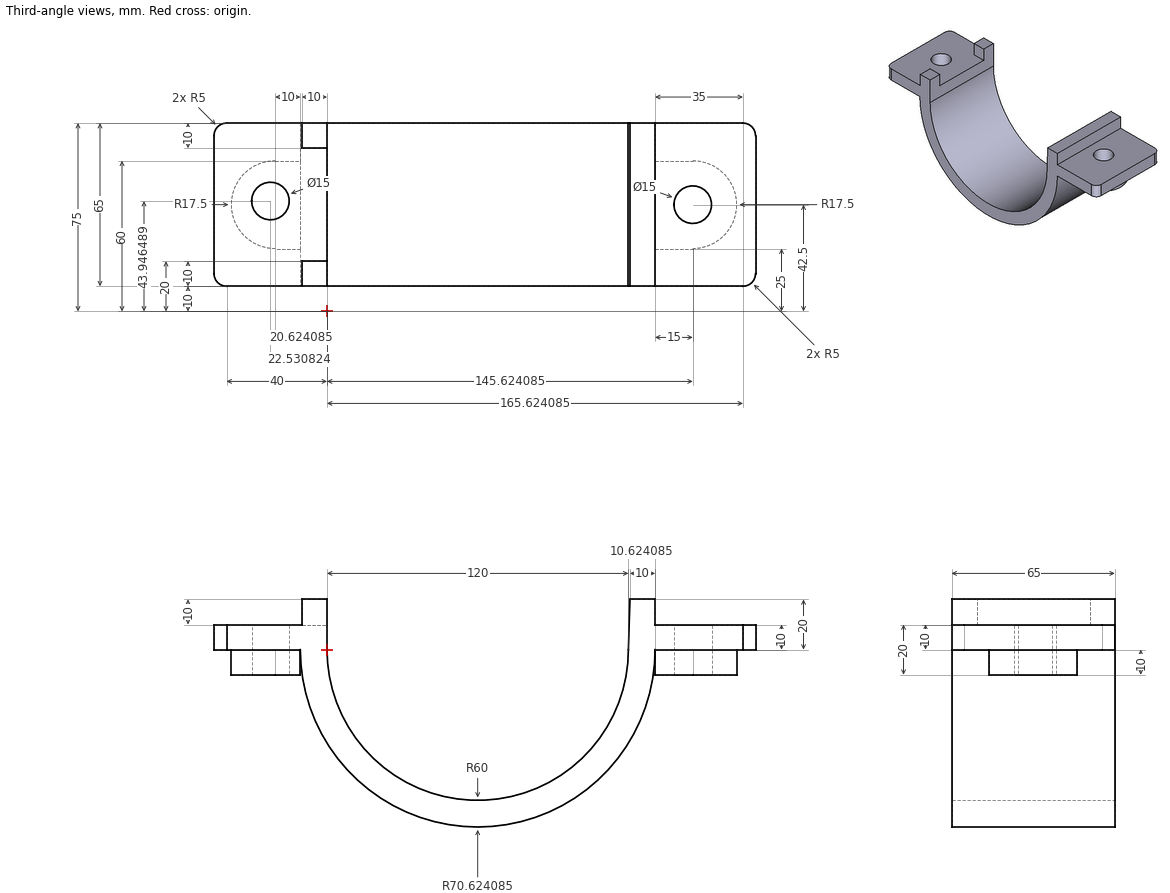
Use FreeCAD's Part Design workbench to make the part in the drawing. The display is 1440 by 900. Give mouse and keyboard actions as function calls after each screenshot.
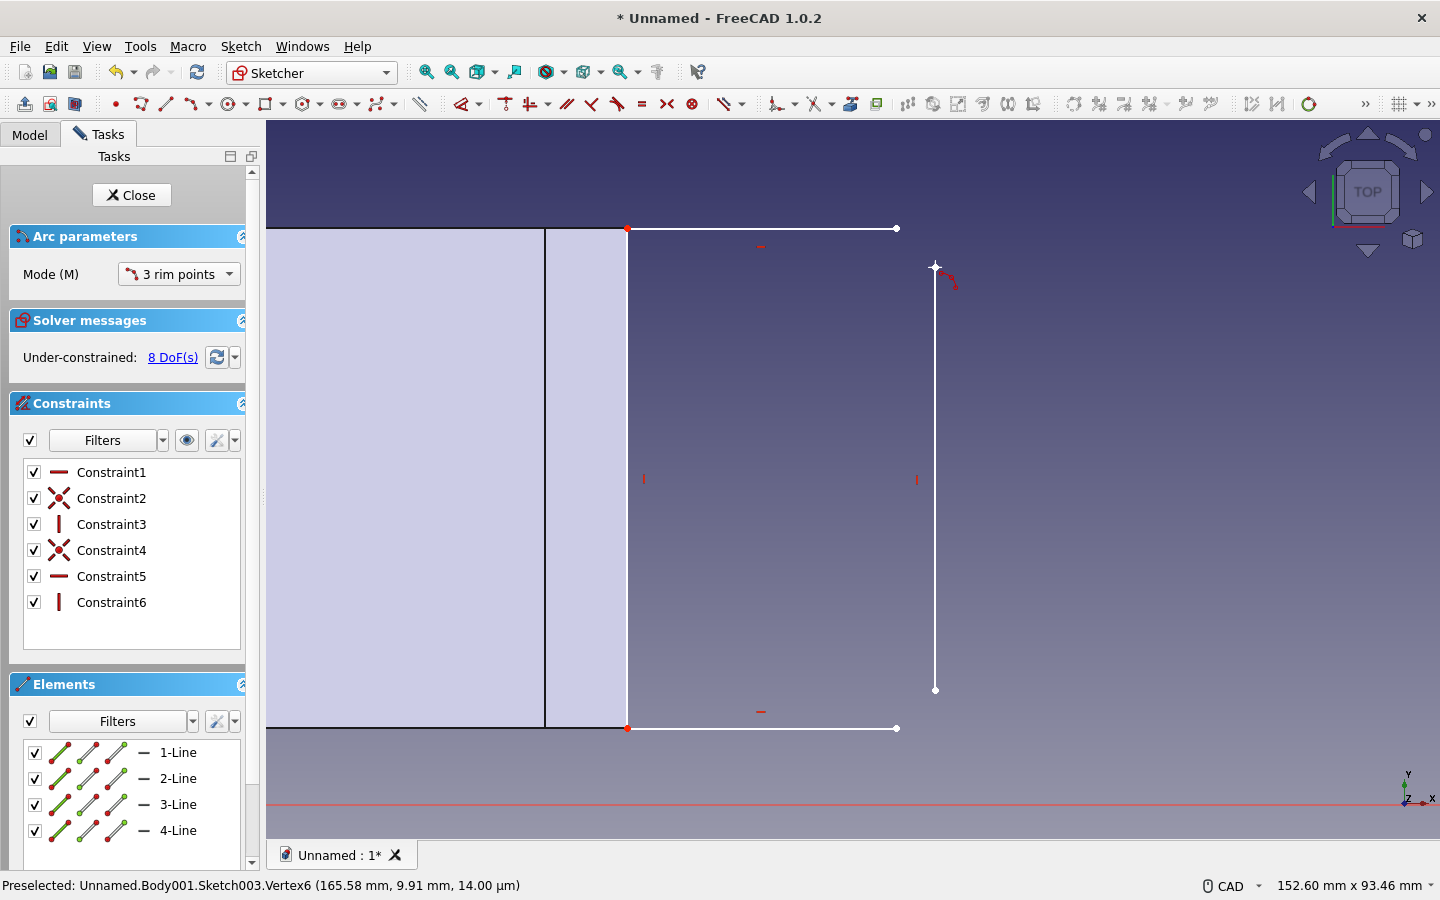
click(896, 729)
click(935, 691)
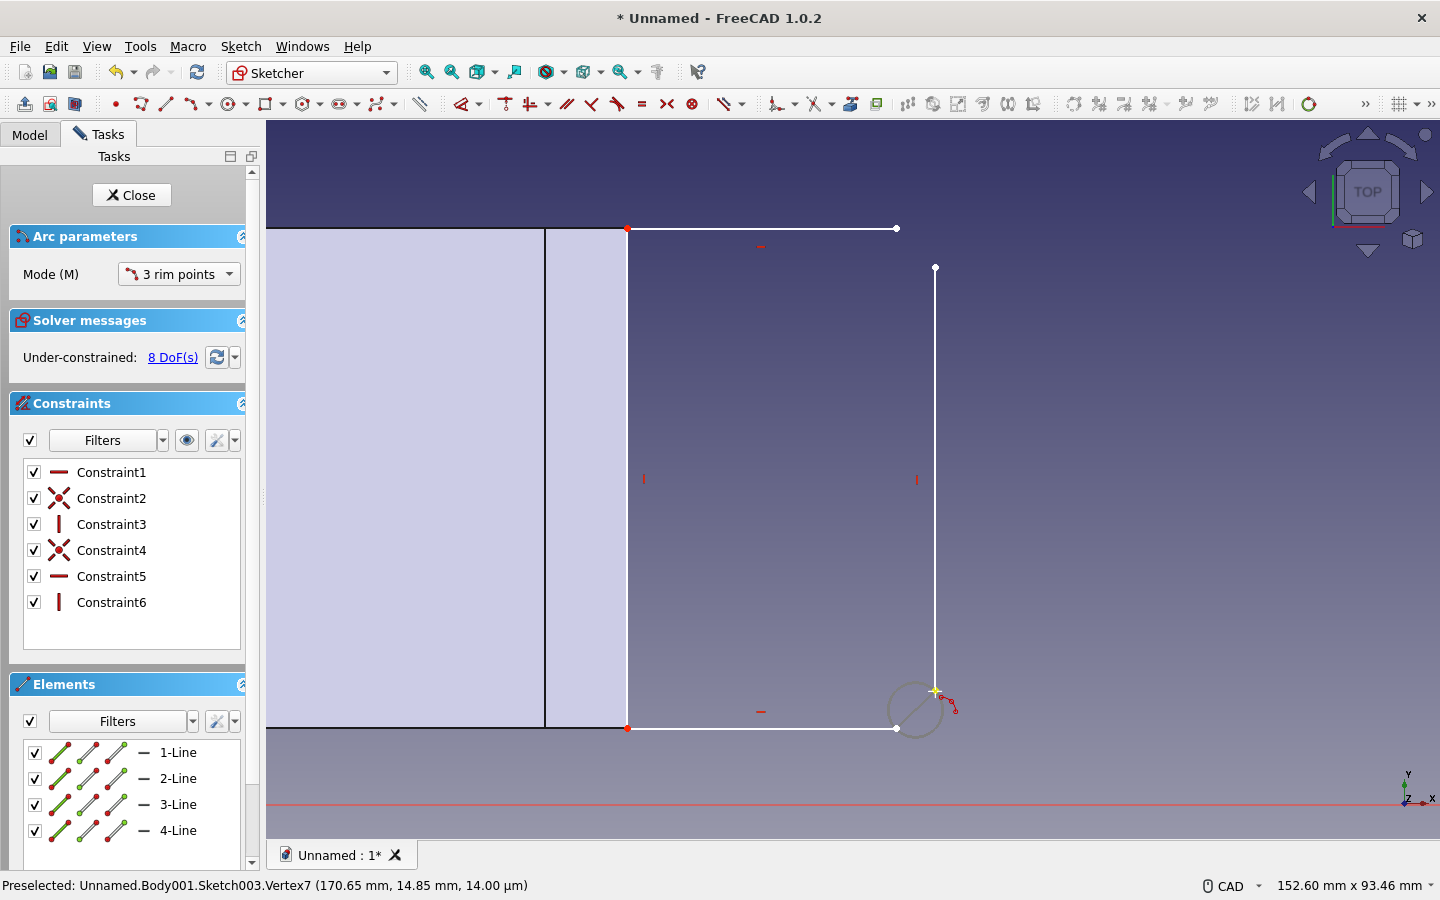
scroll(924, 717, up, 2)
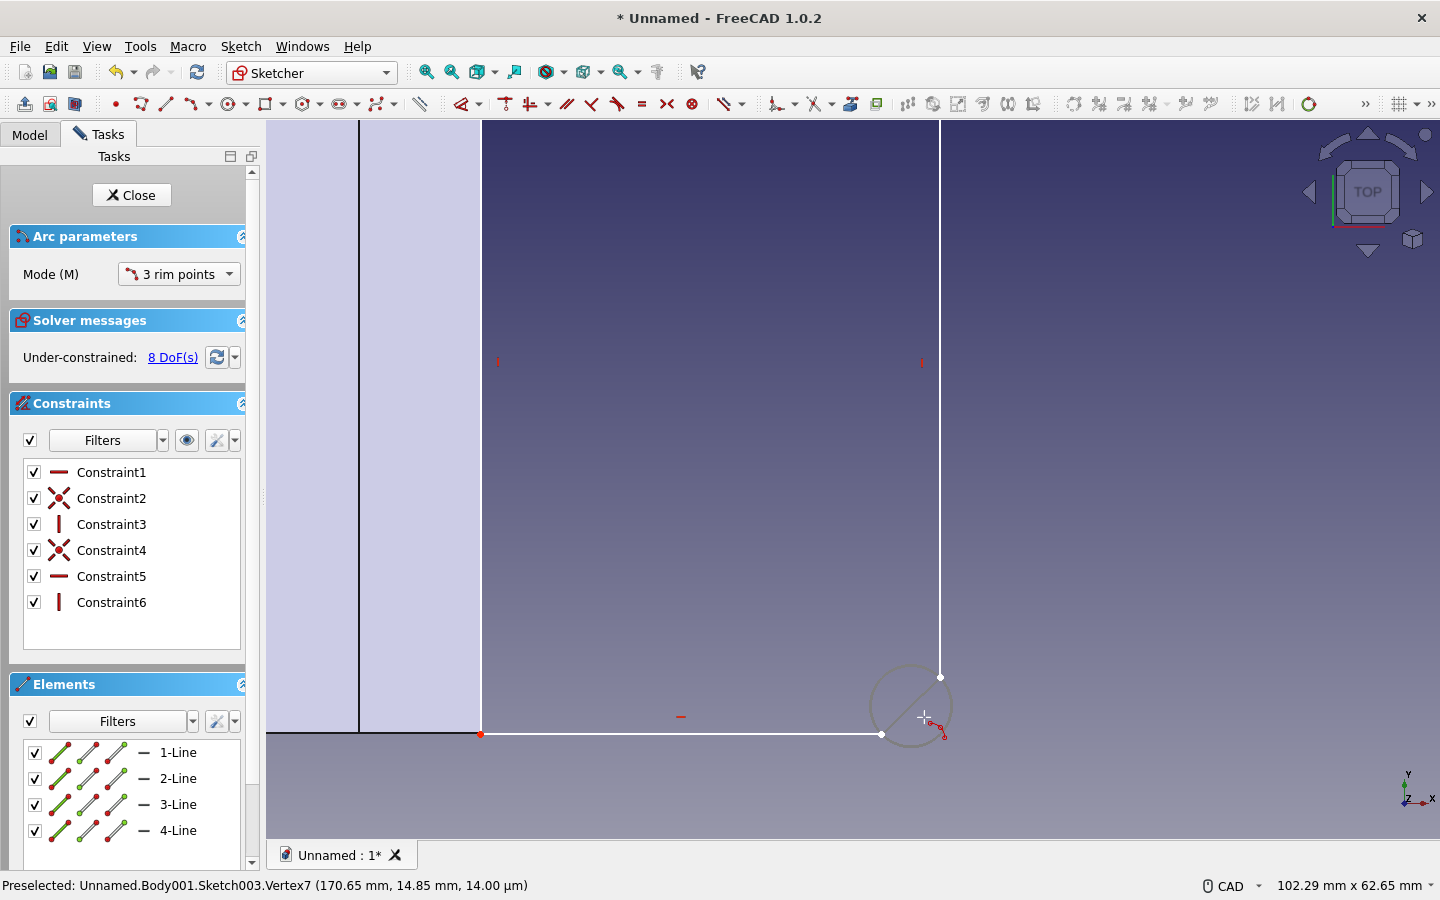
click(923, 717)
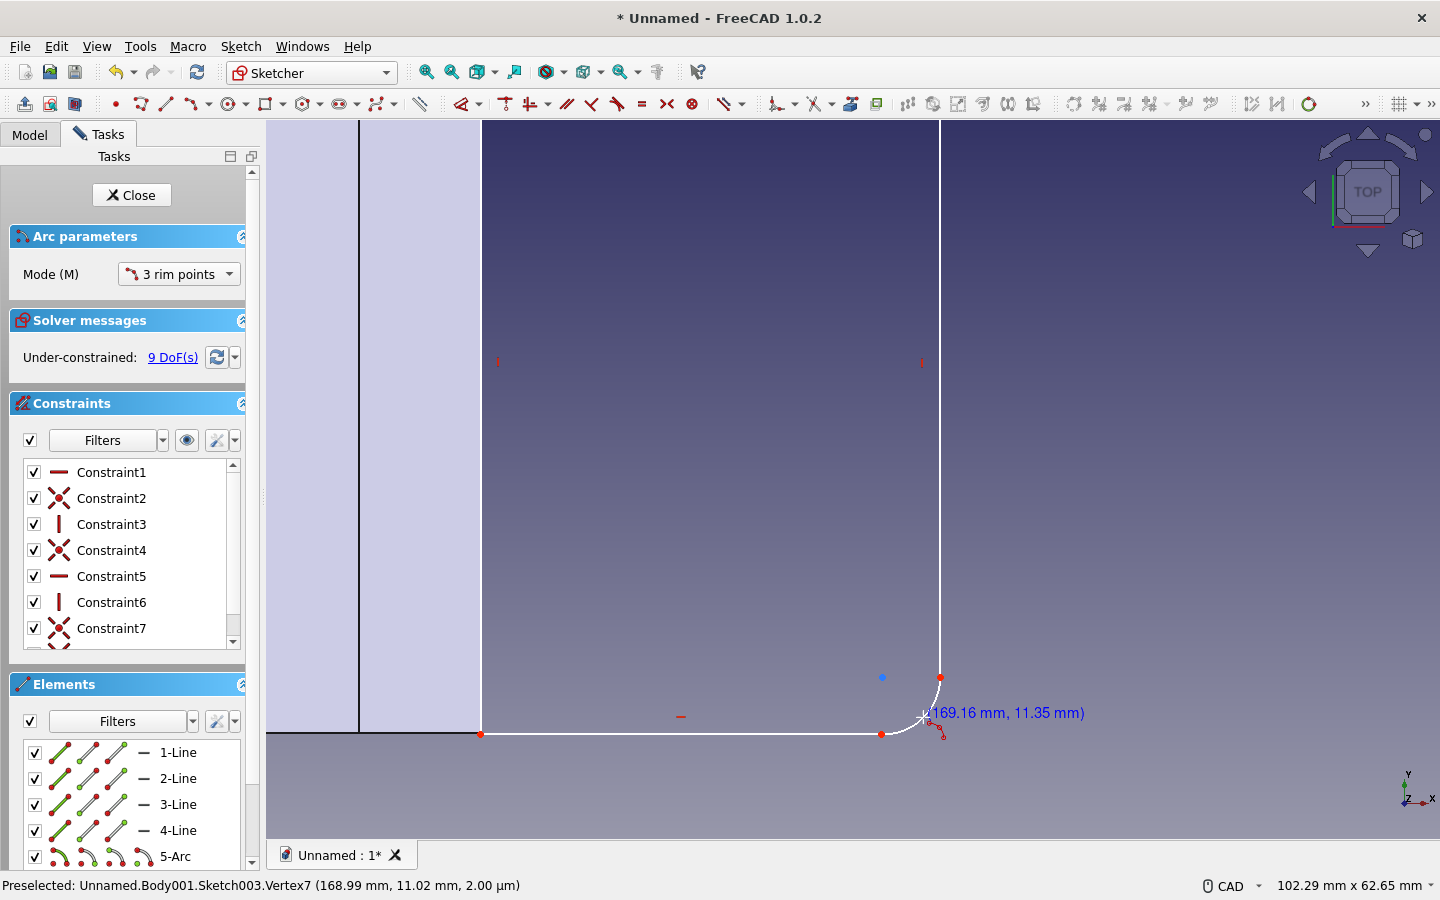
scroll(935, 722, down, 2)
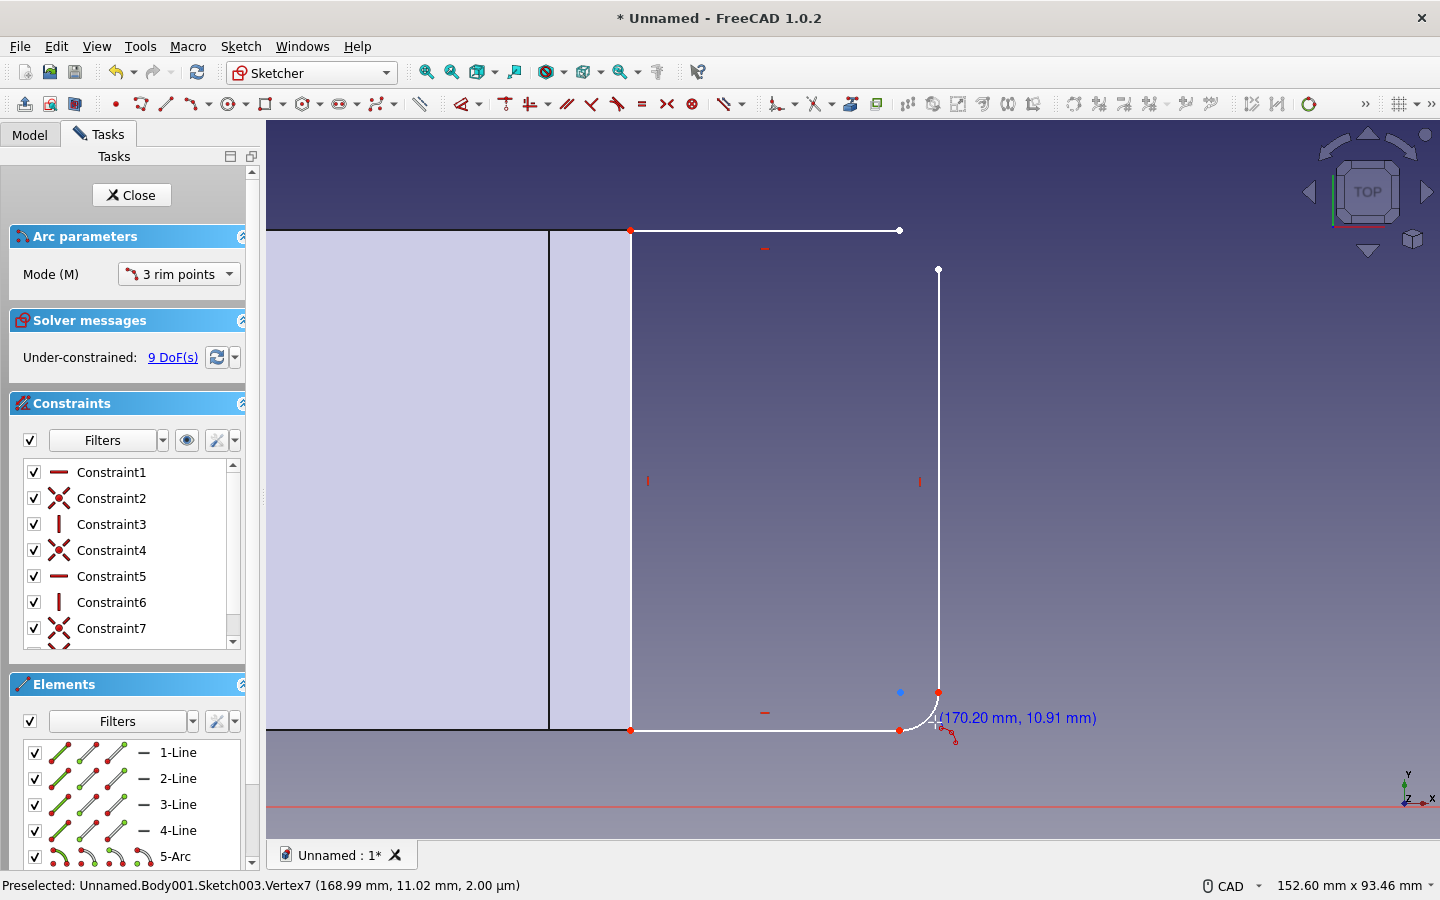
click(939, 270)
click(900, 231)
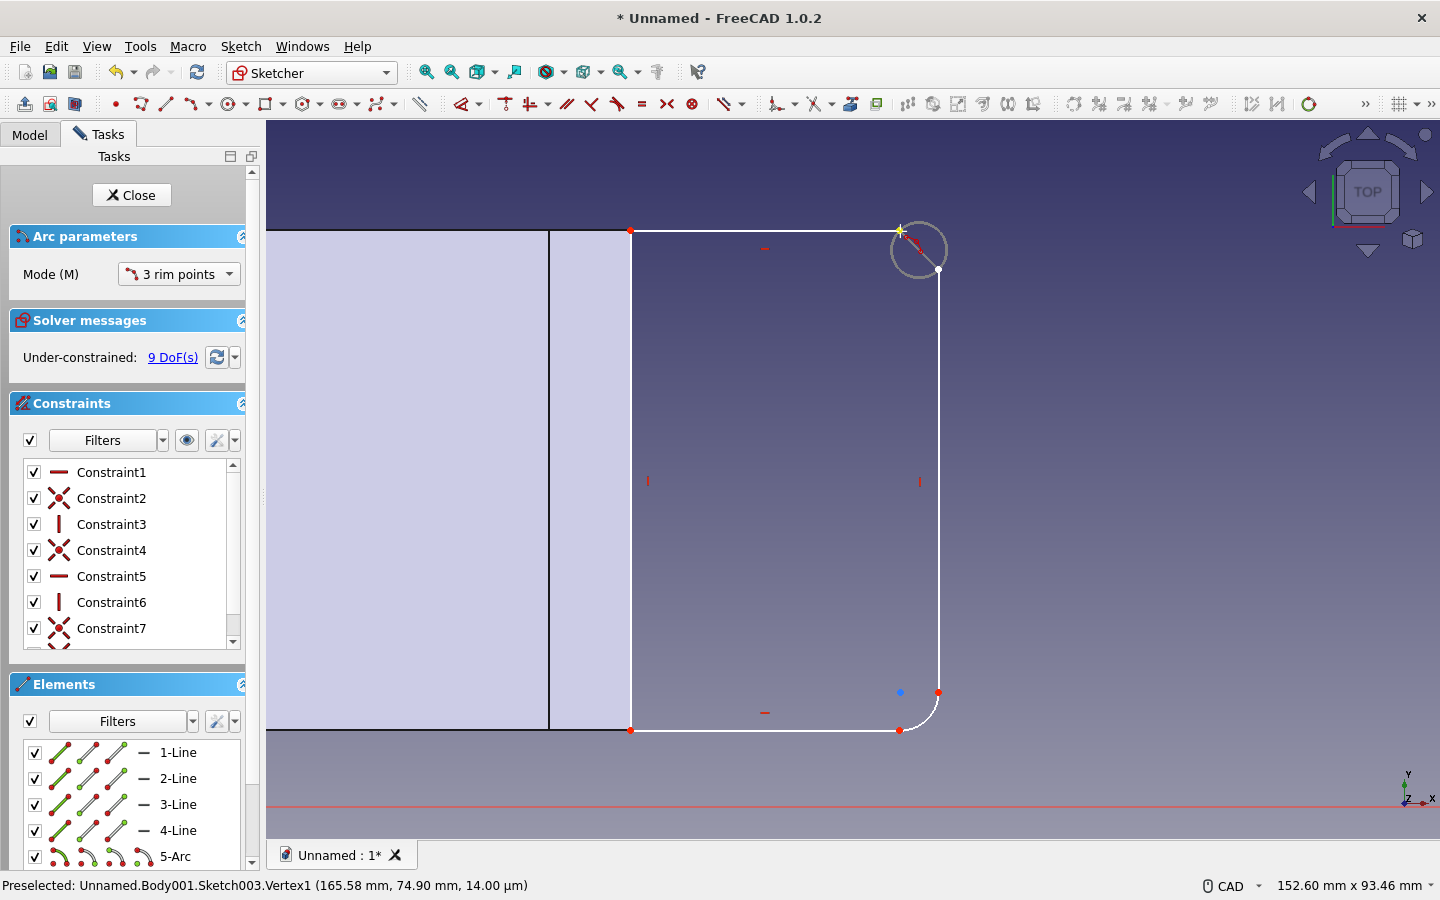
scroll(927, 241, up, 2)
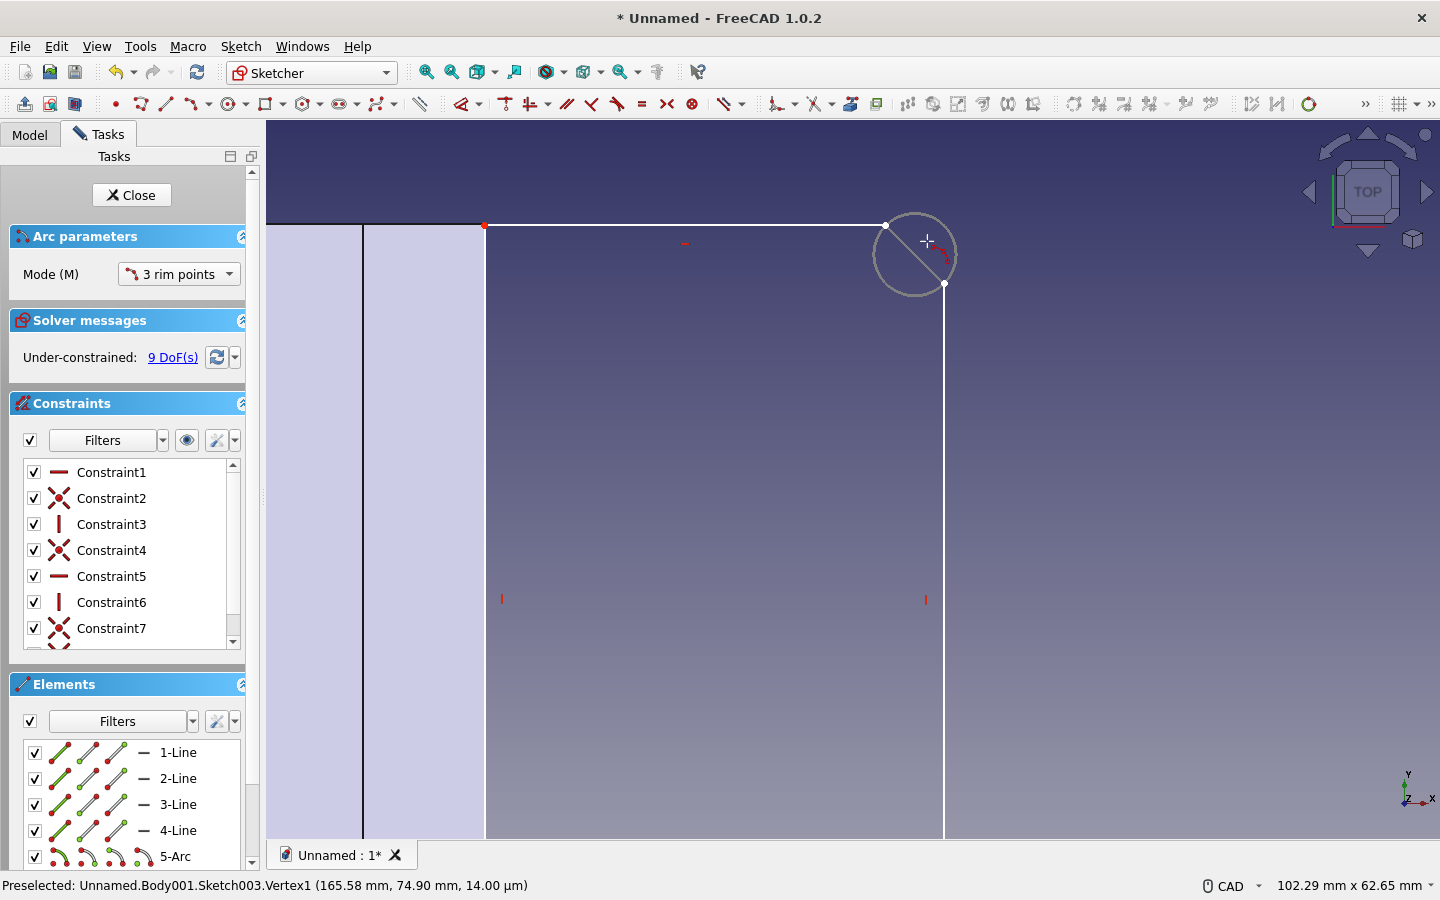
click(927, 241)
key(Escape)